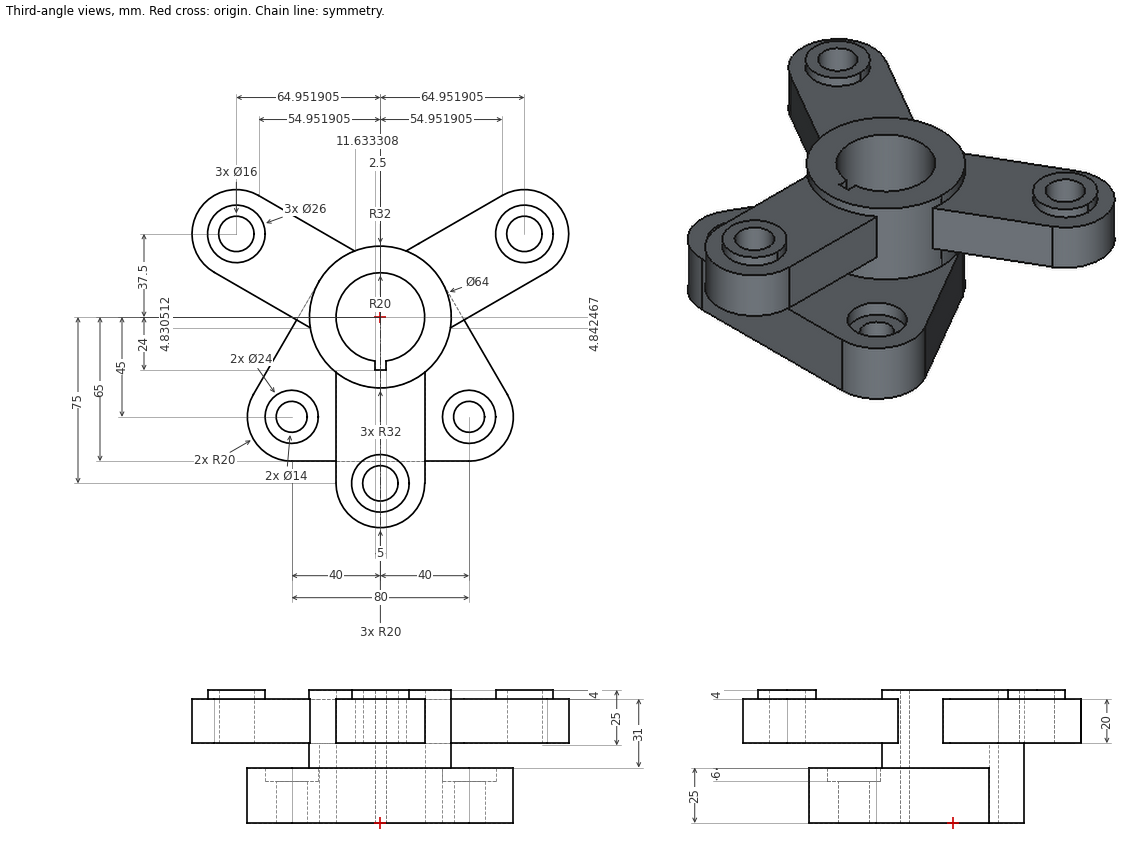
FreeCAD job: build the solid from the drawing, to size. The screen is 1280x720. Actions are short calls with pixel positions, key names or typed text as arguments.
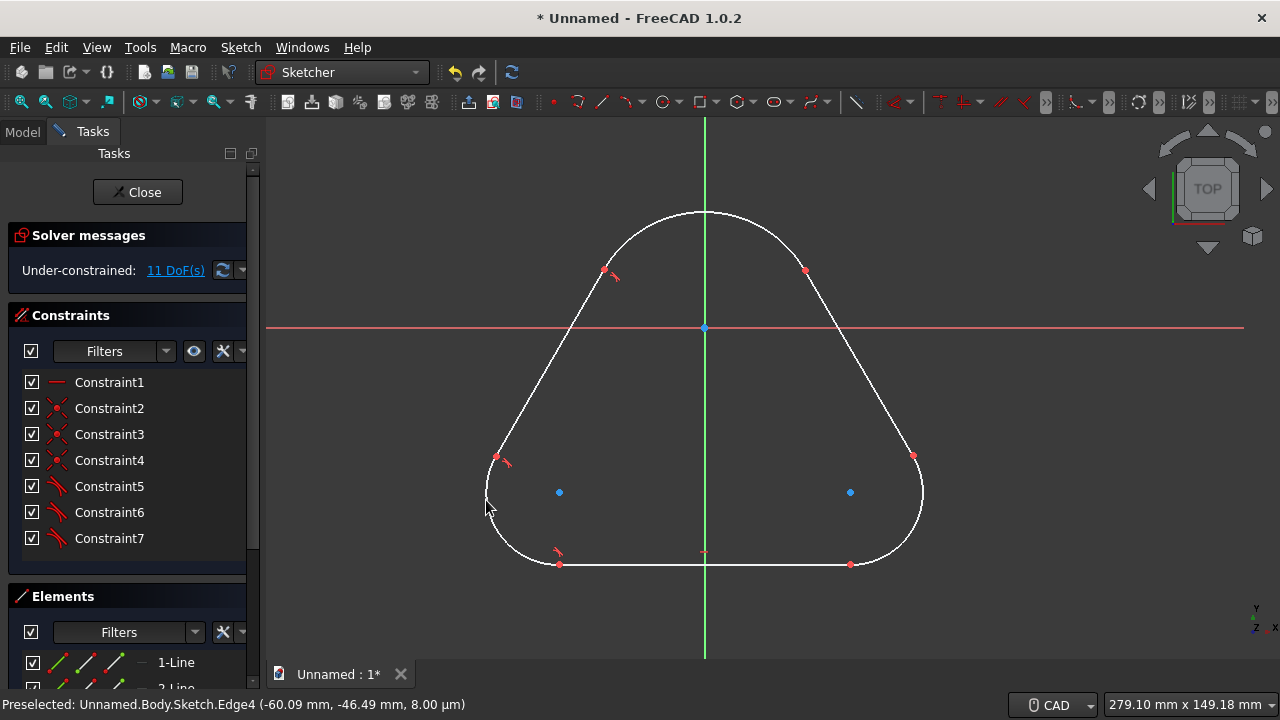
click(646, 565)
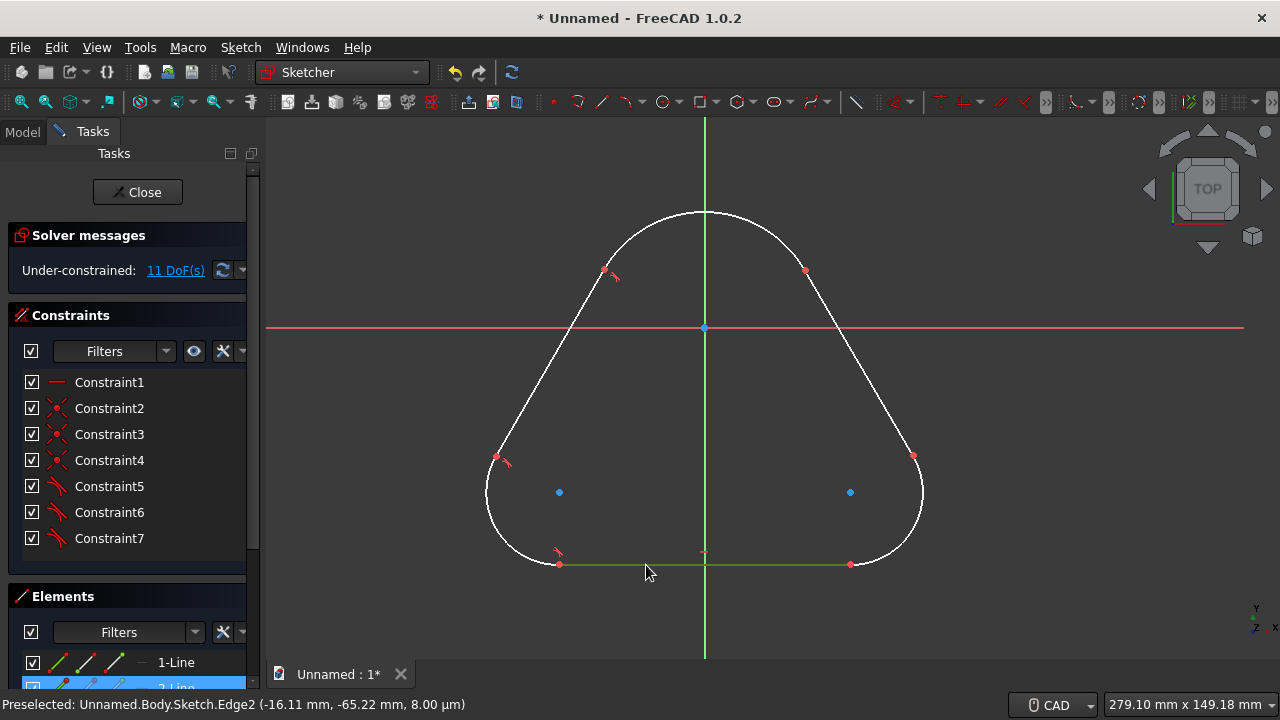
click(893, 551)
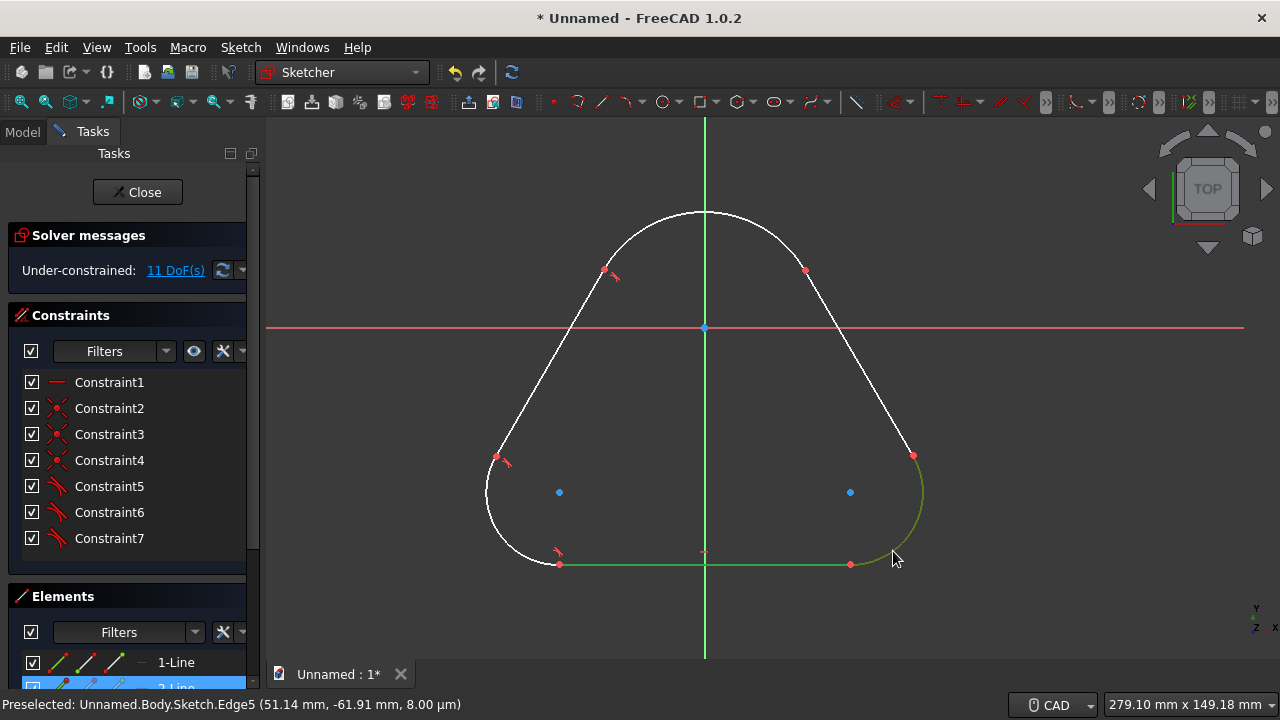
key(t)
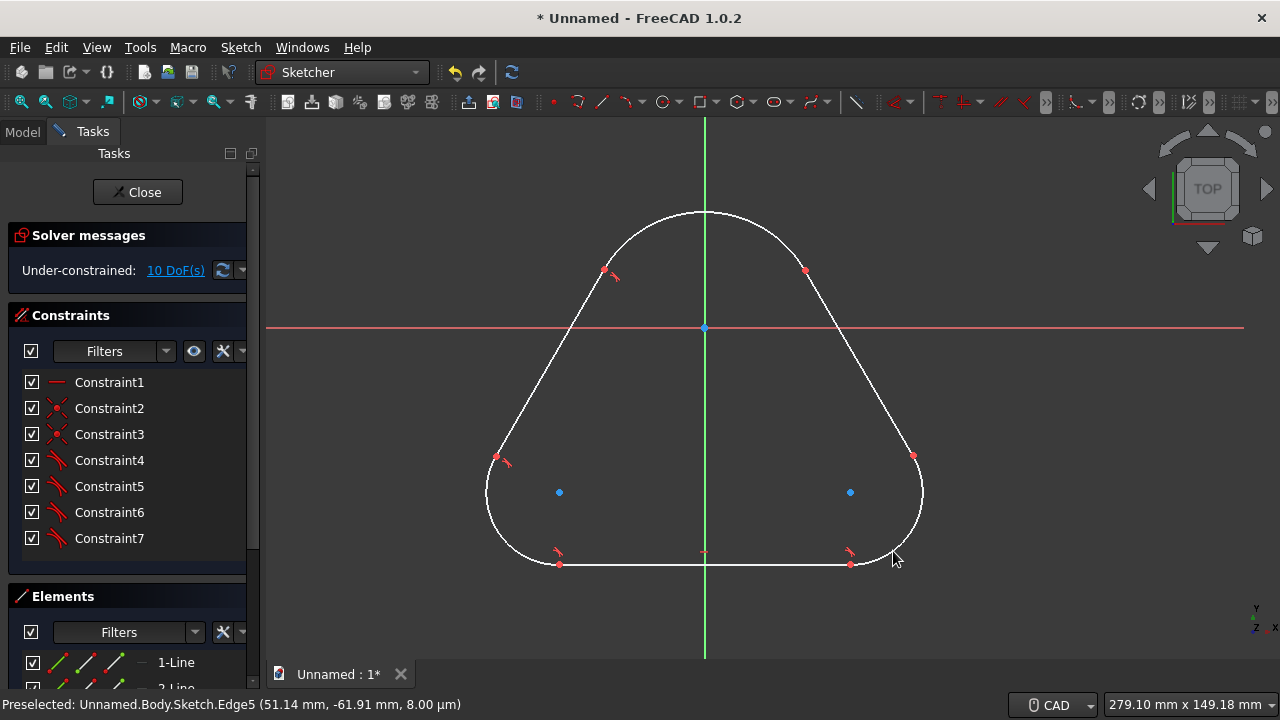
click(881, 401)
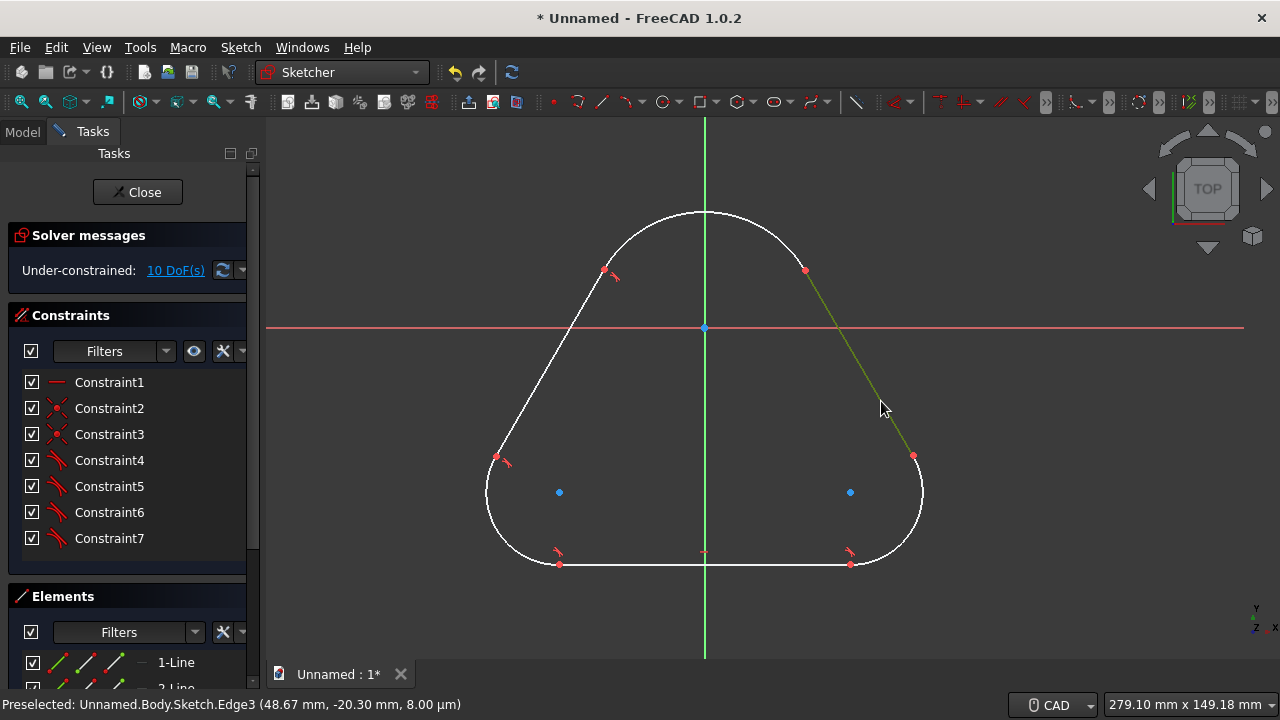
click(893, 551)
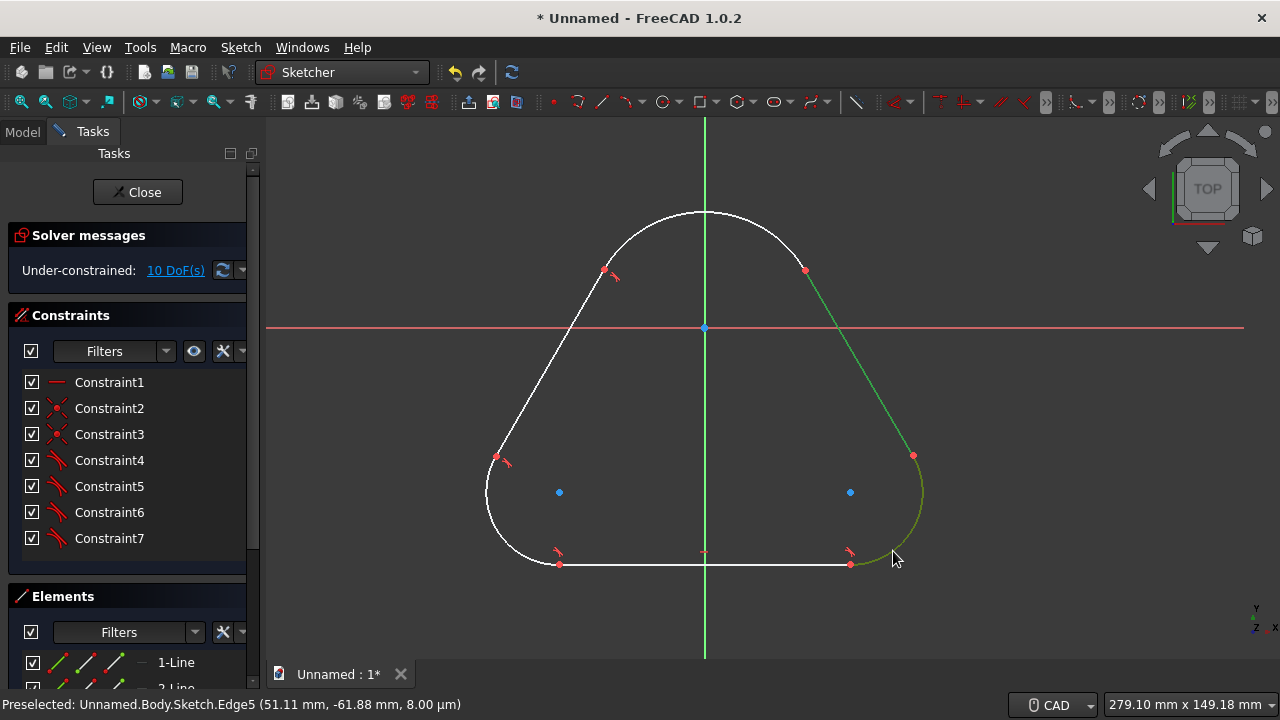
key(t)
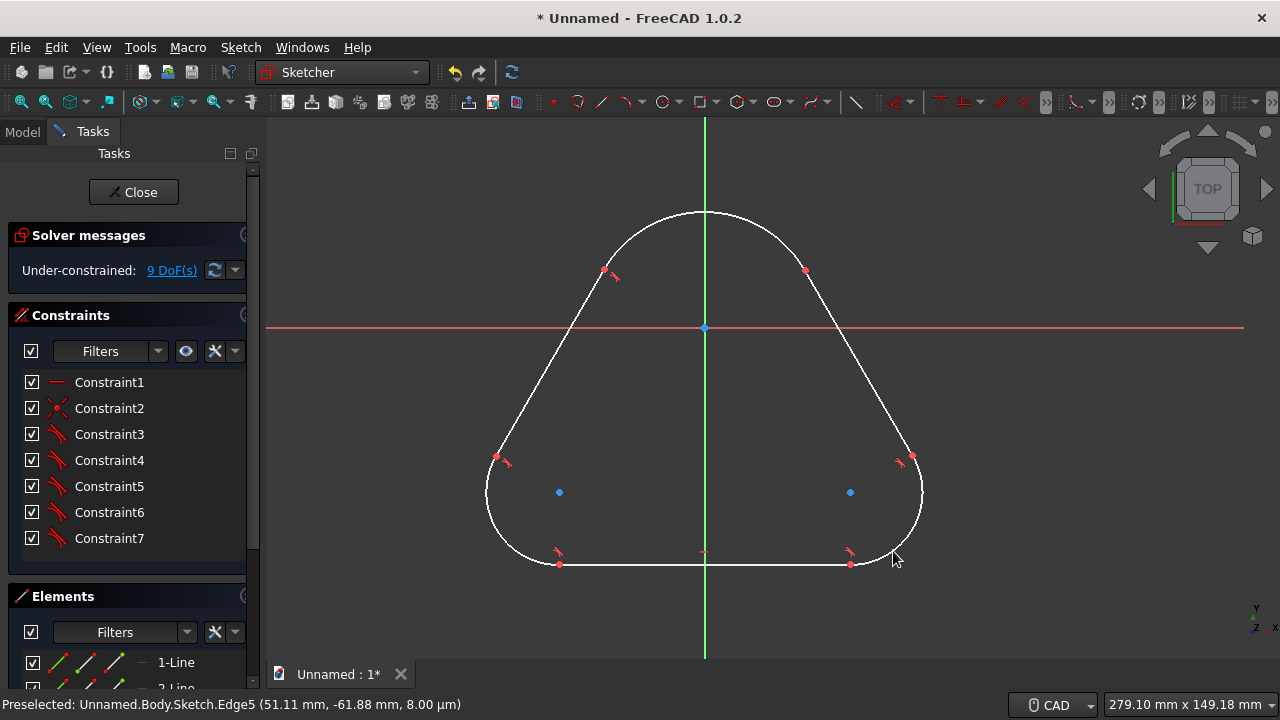
click(880, 400)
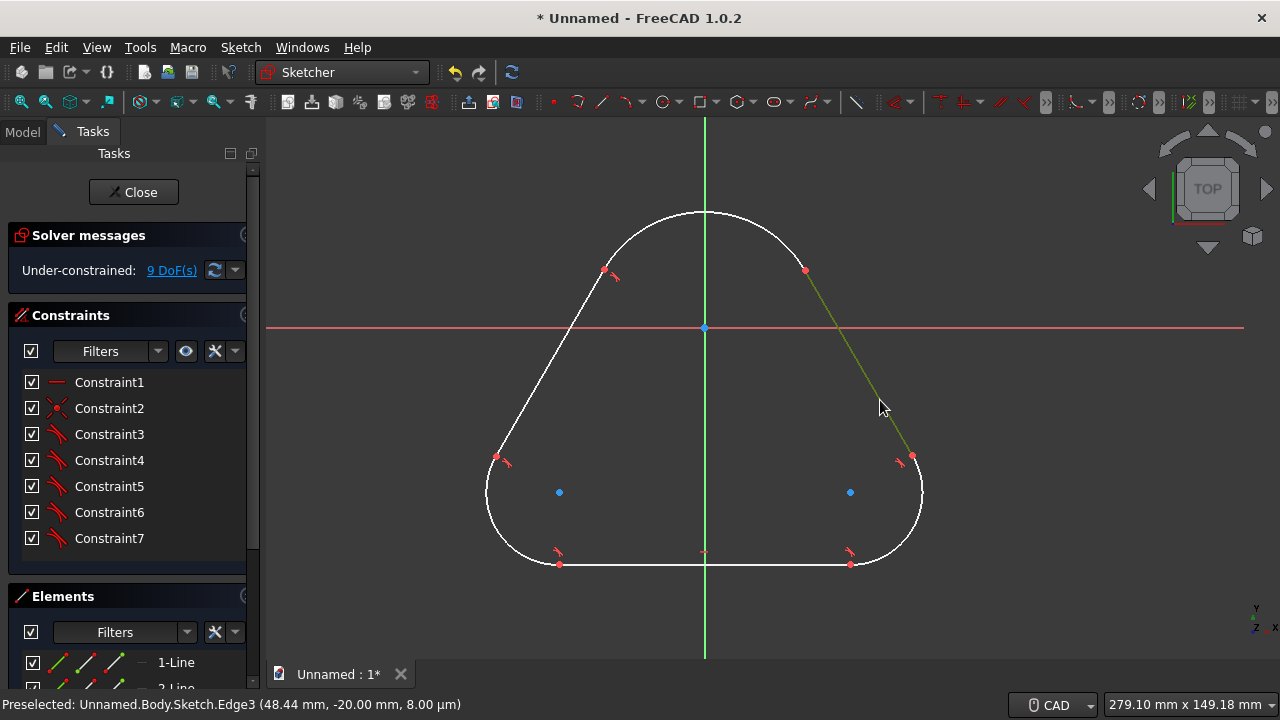
click(752, 222)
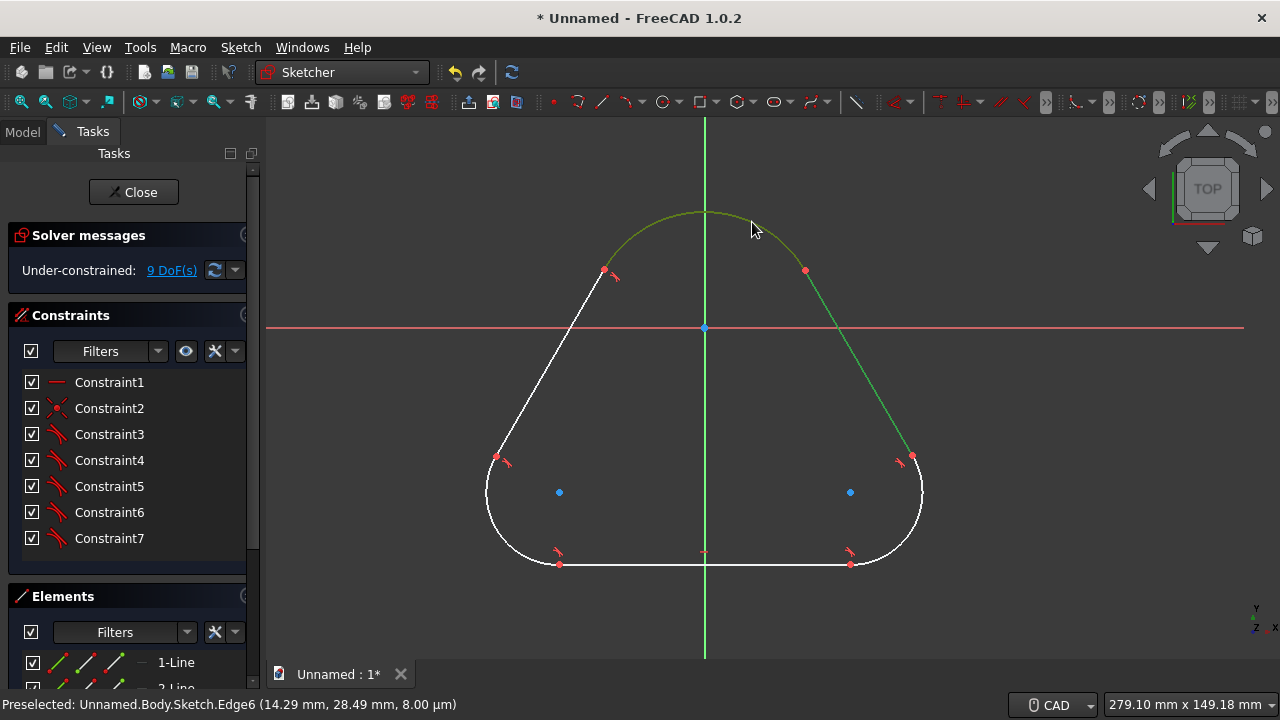
key(t)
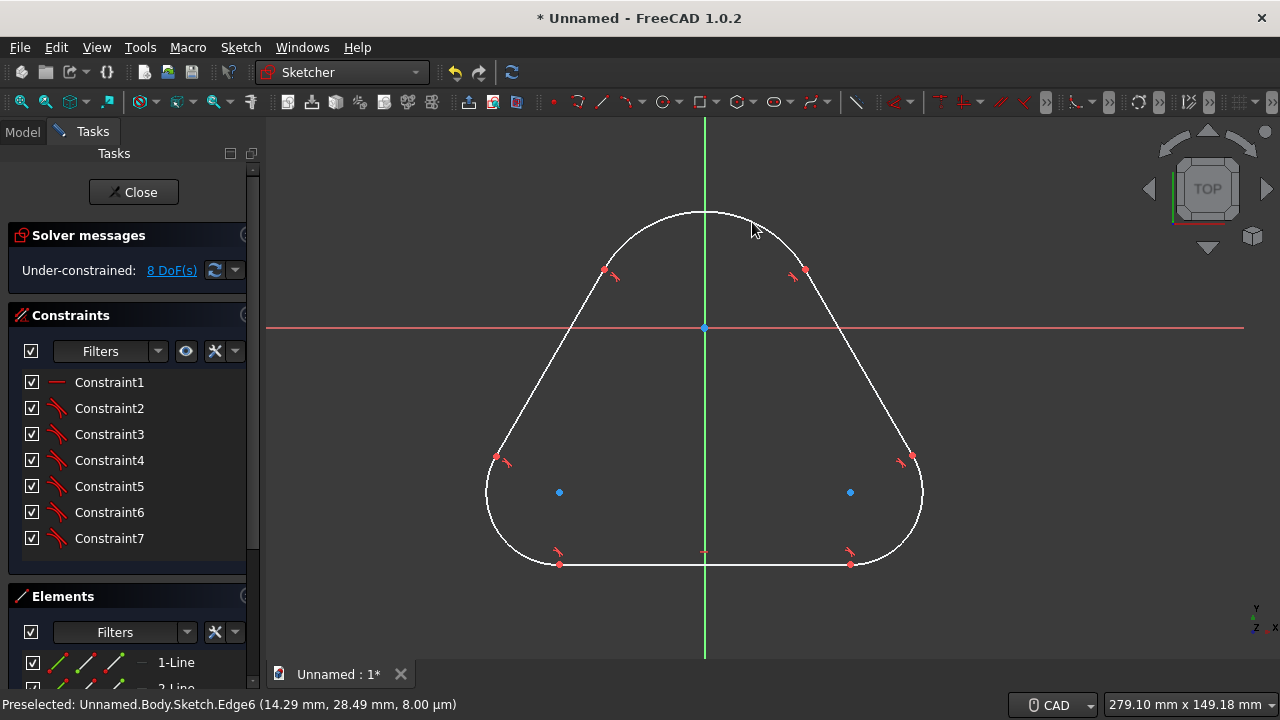
drag(695, 318, 715, 338)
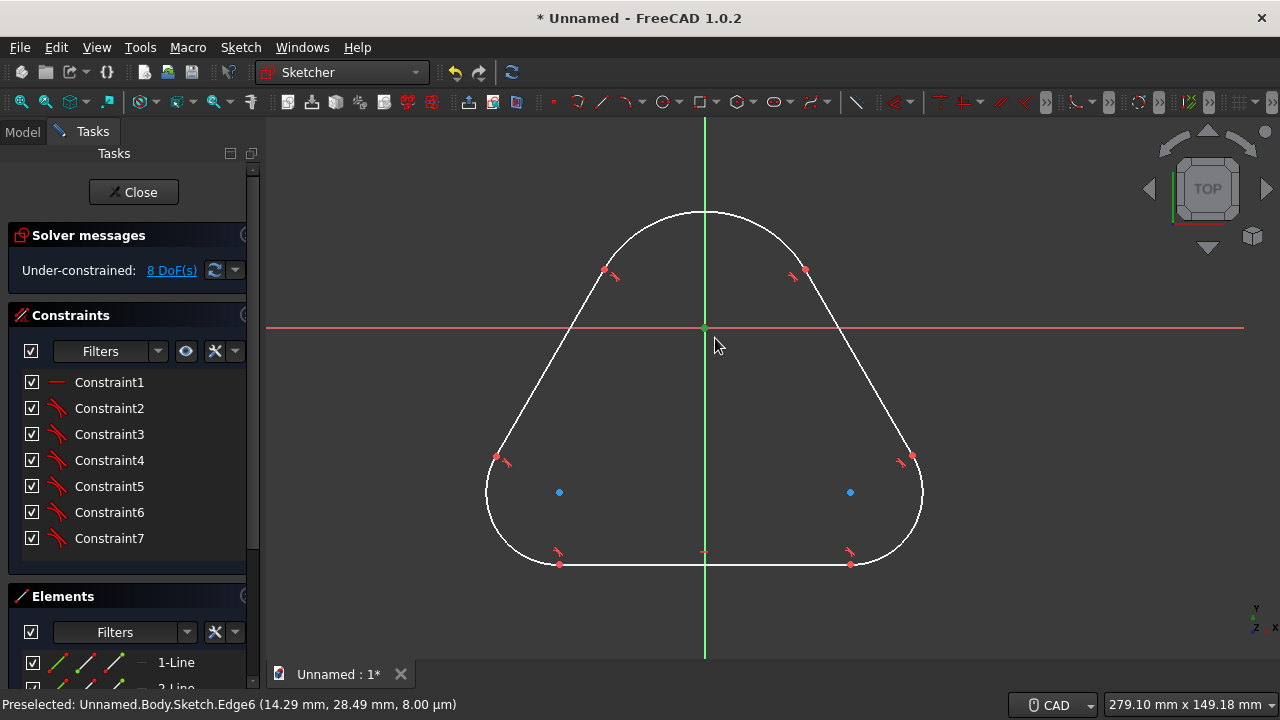
click(940, 102)